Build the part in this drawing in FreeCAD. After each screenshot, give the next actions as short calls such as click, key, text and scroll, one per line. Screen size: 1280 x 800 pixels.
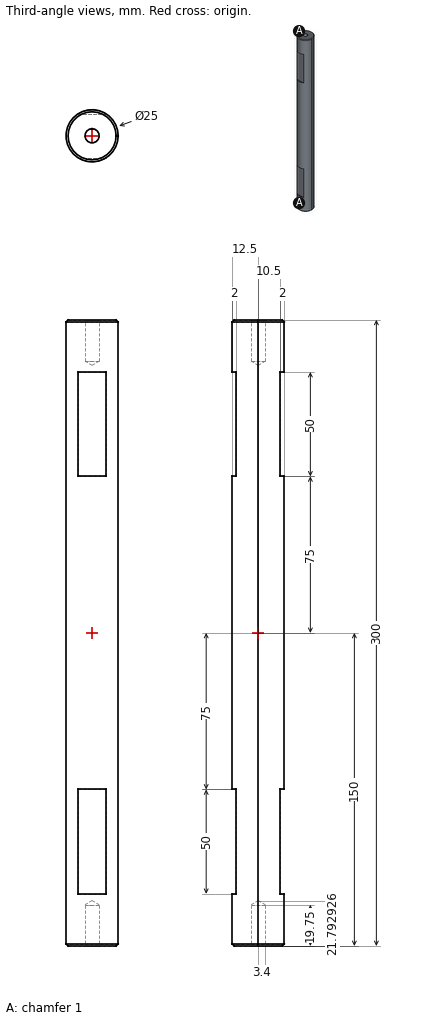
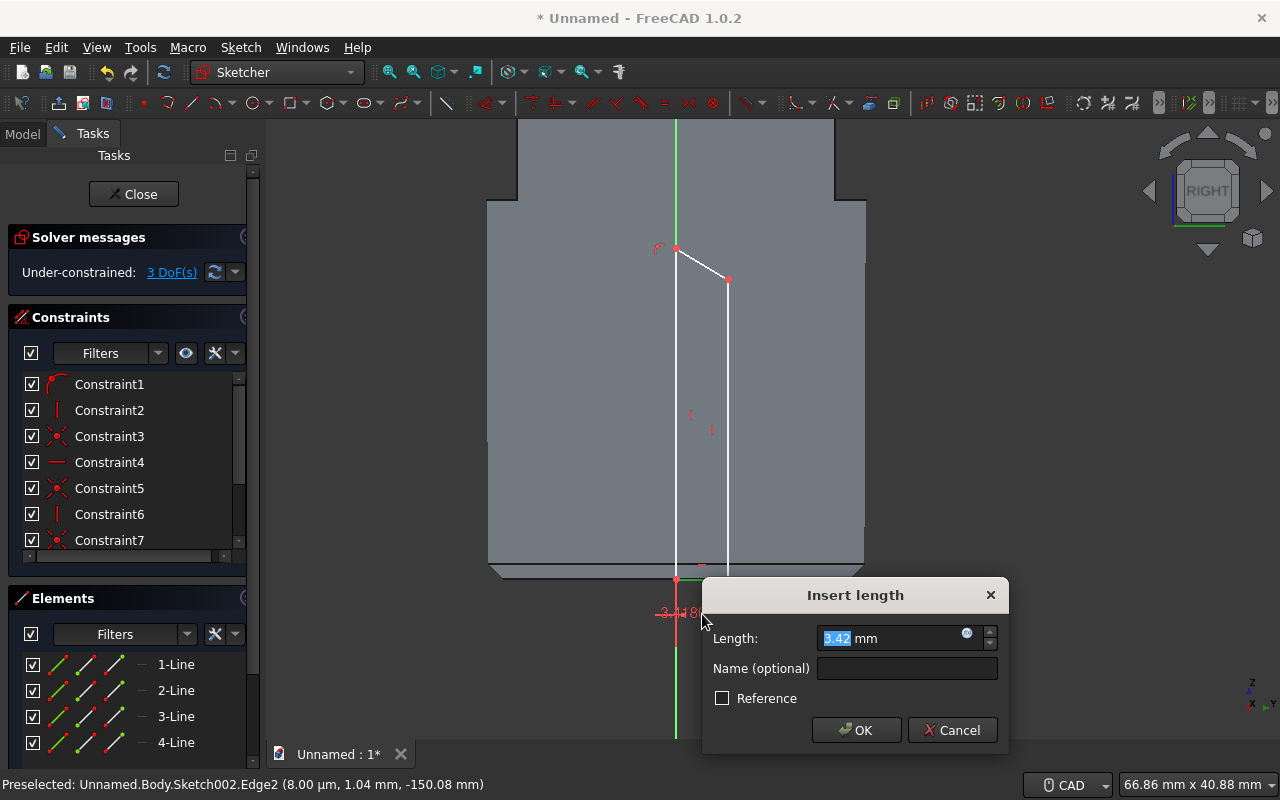
text(3.4)
key(Return)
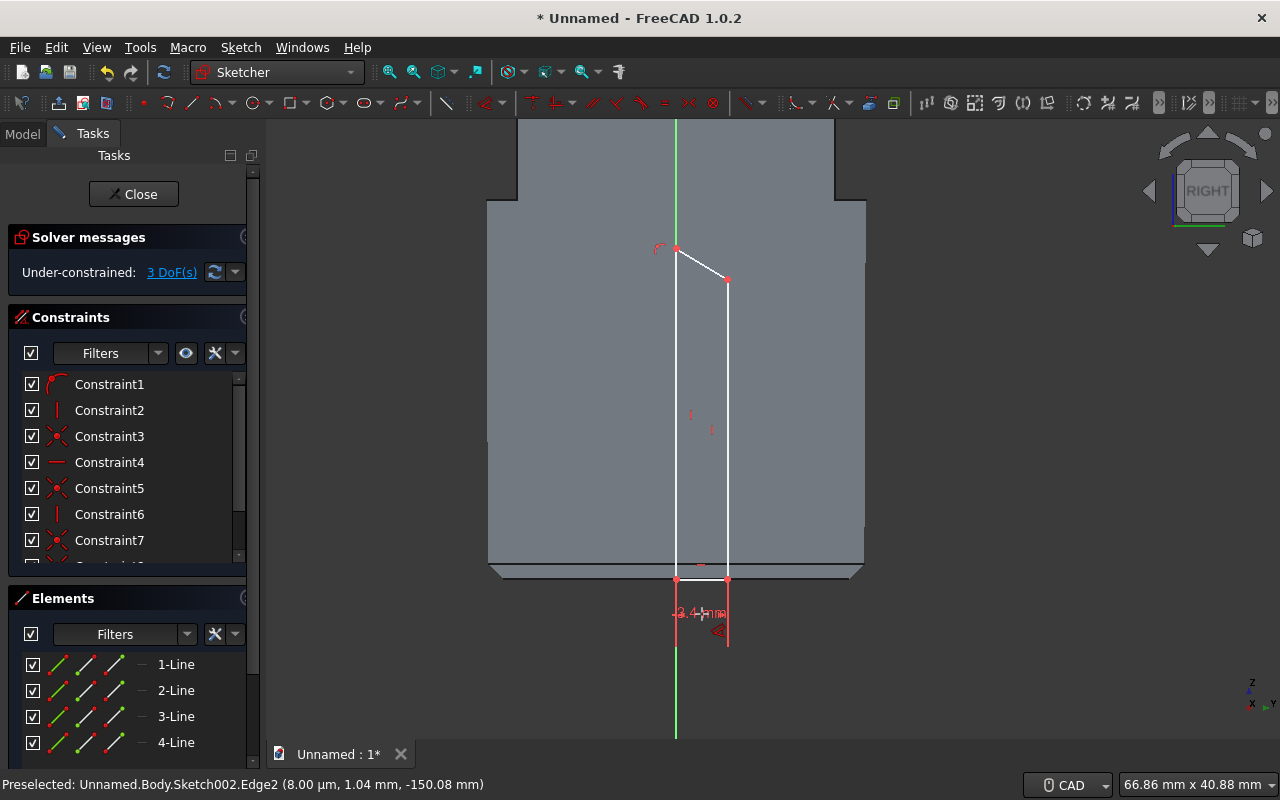
click(676, 580)
click(642, 364)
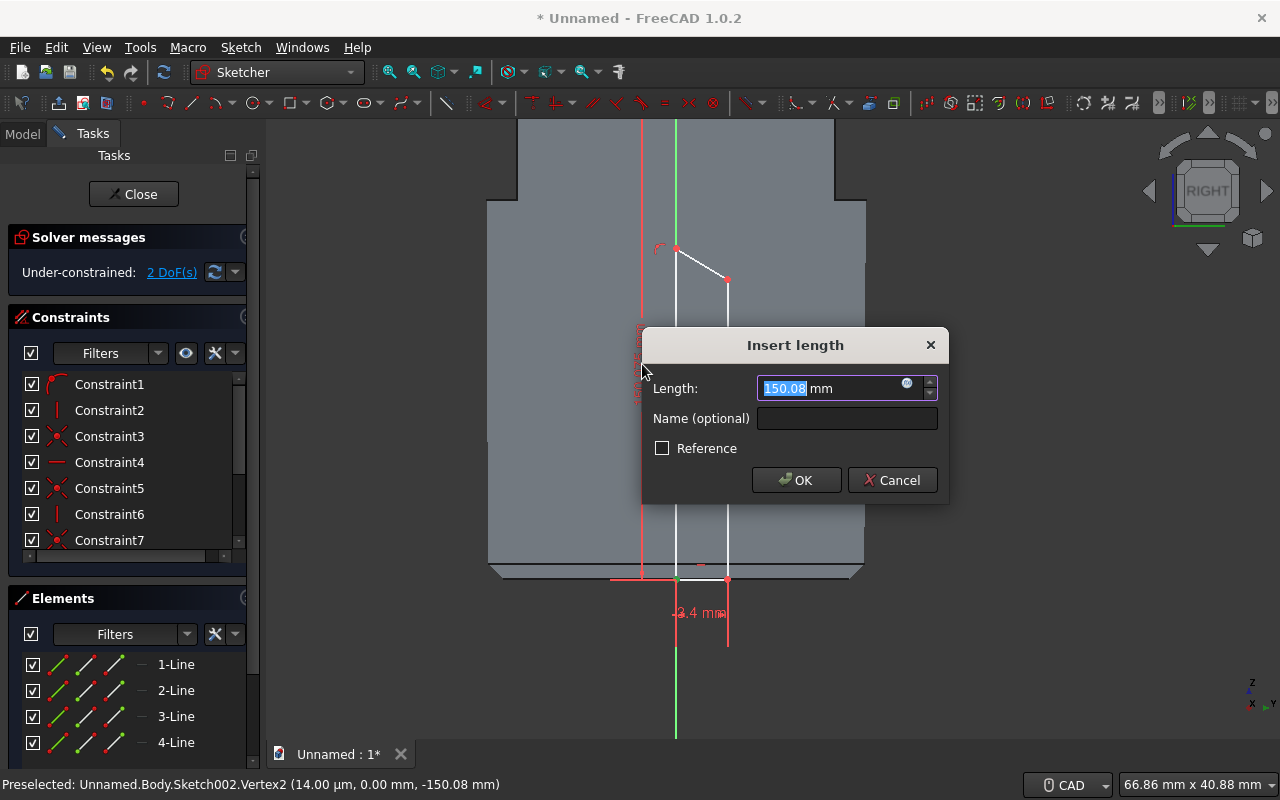
text(150)
key(Return)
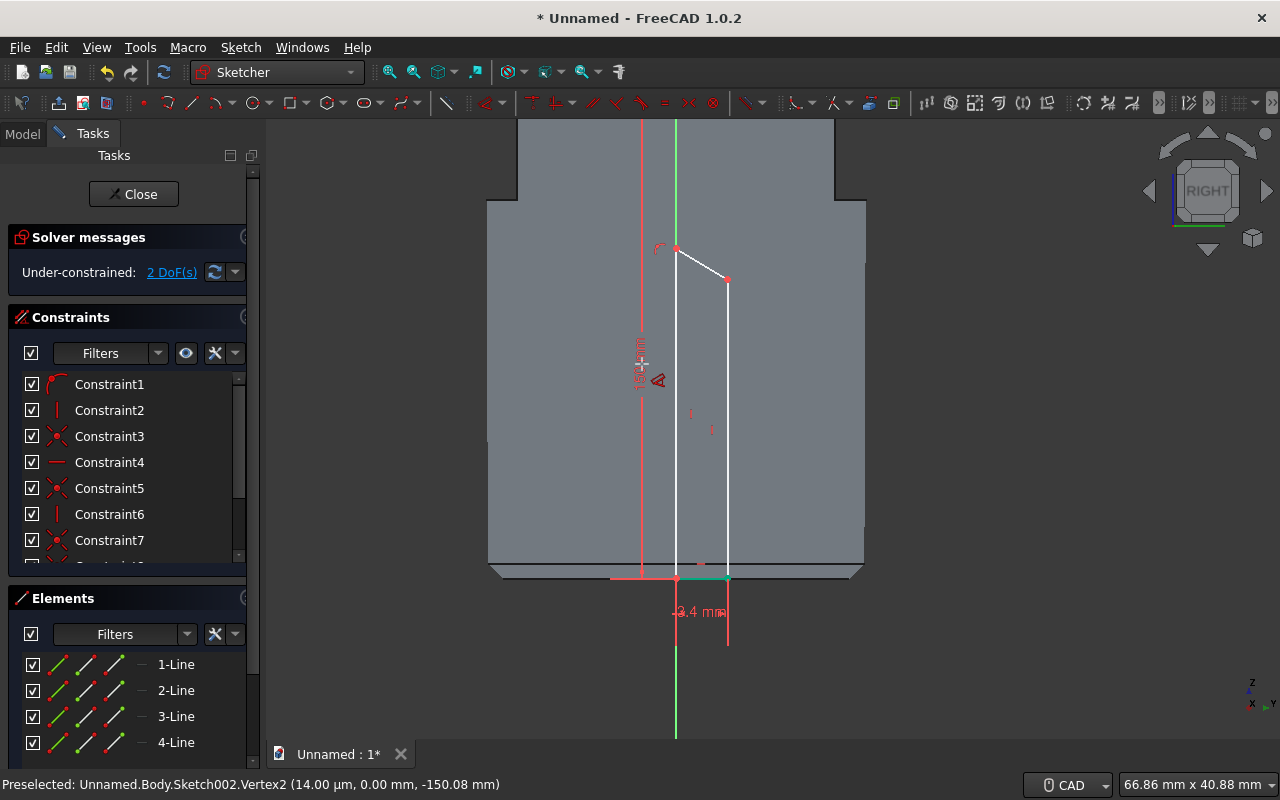
click(728, 489)
click(762, 429)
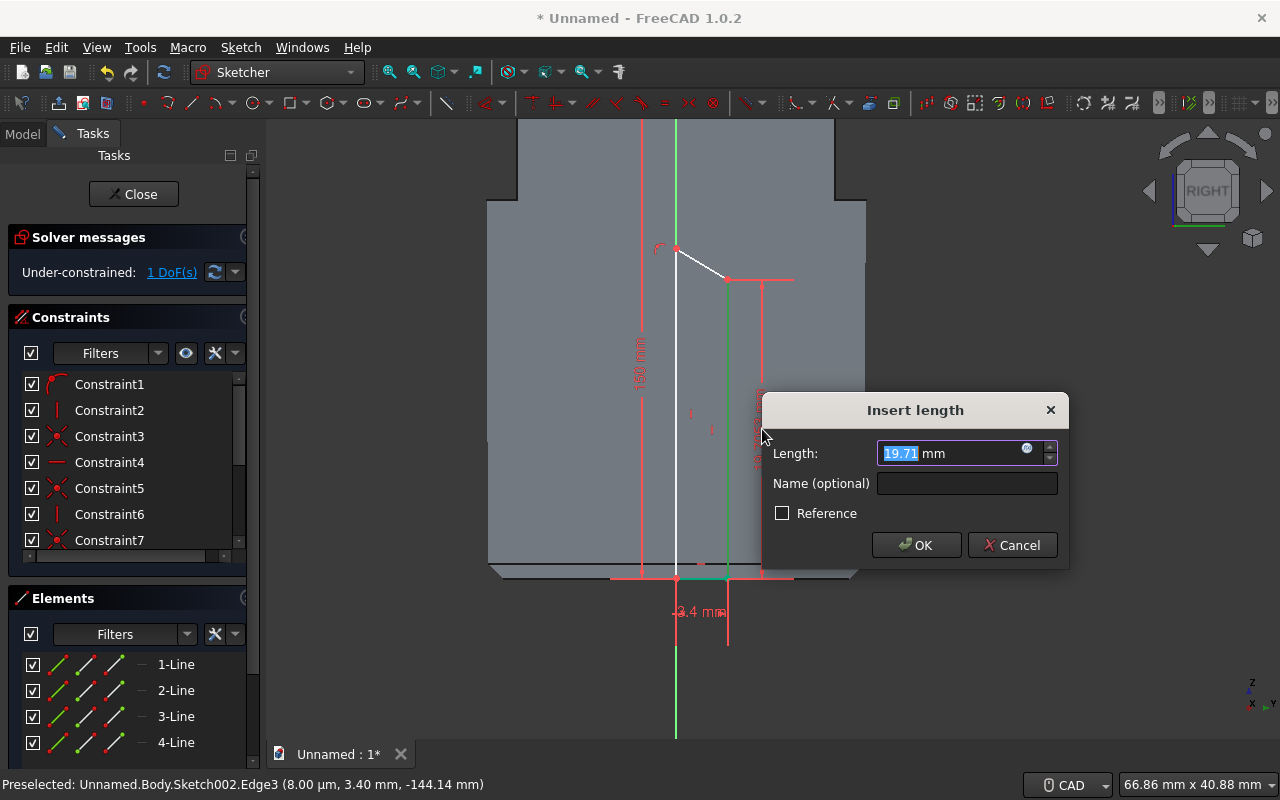
text(19.75)
key(Return)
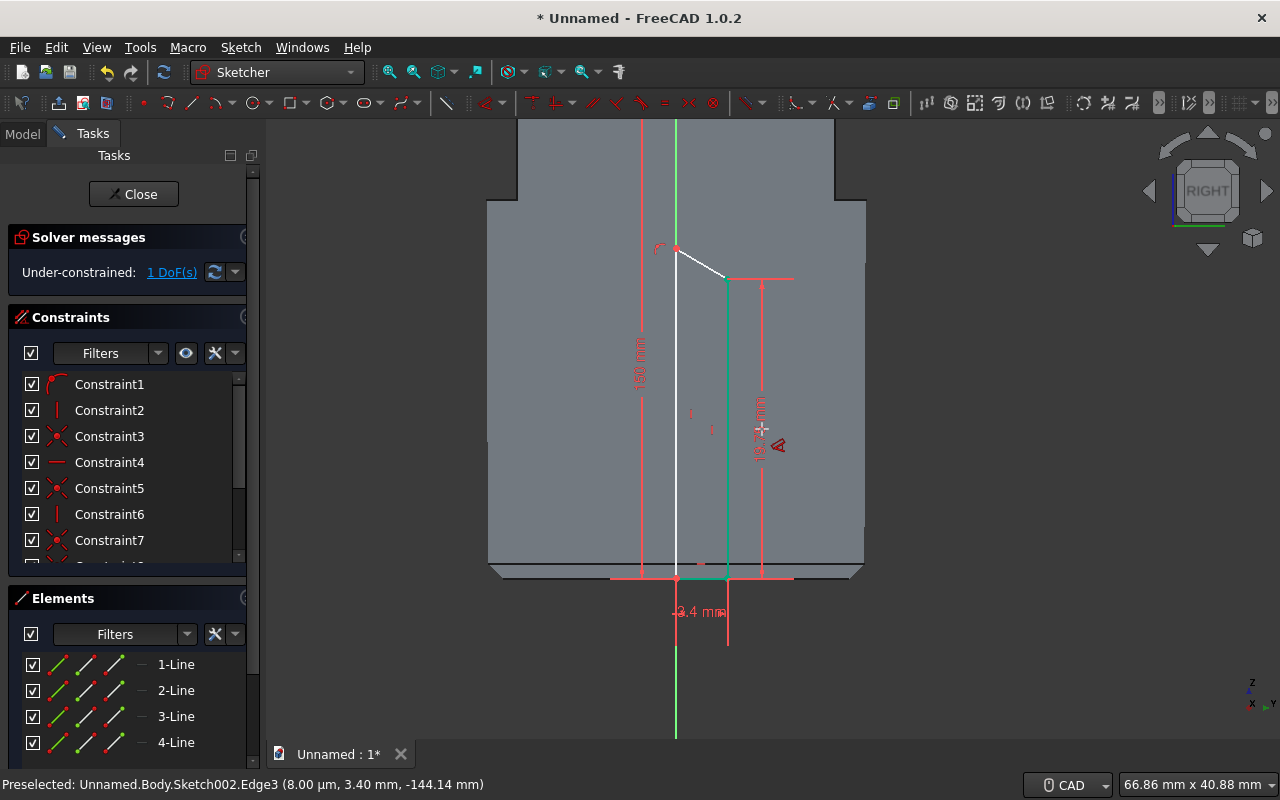
click(676, 348)
click(642, 414)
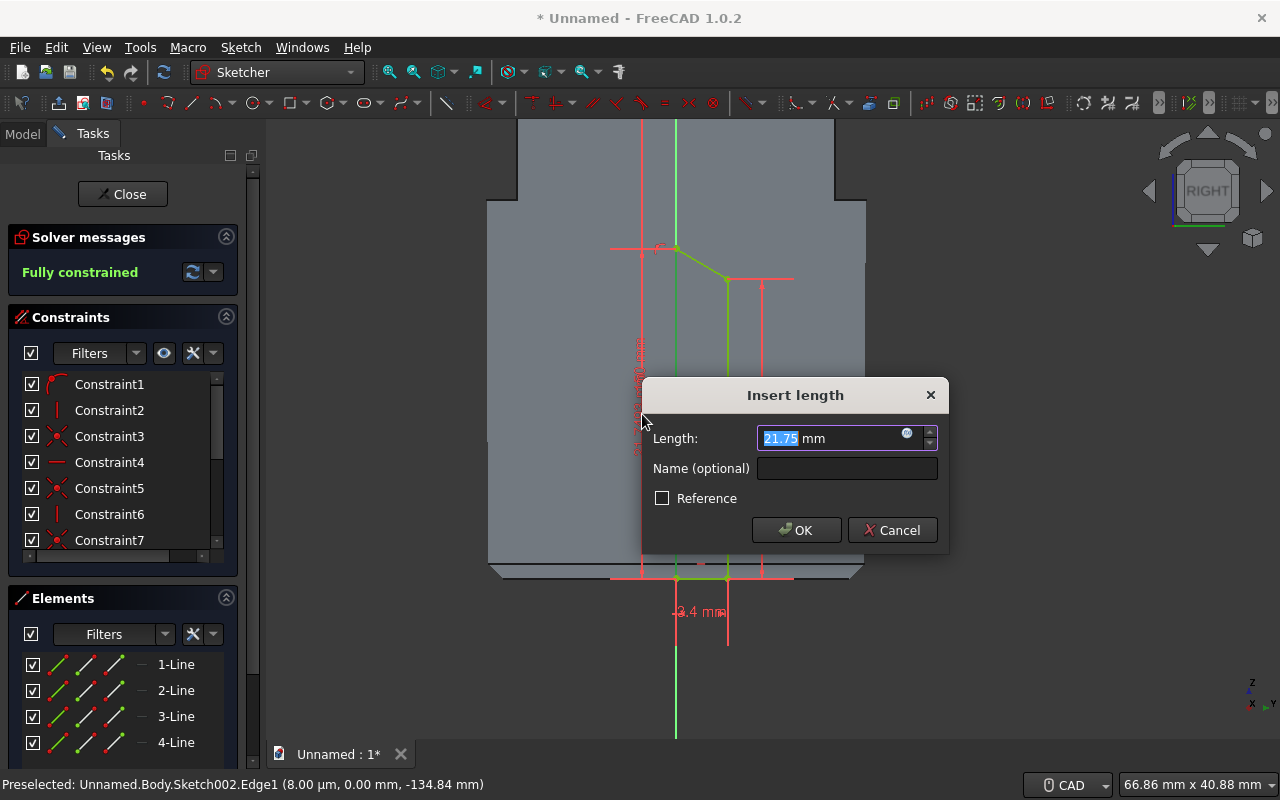
text(21.792926)
key(Return)
key(Escape)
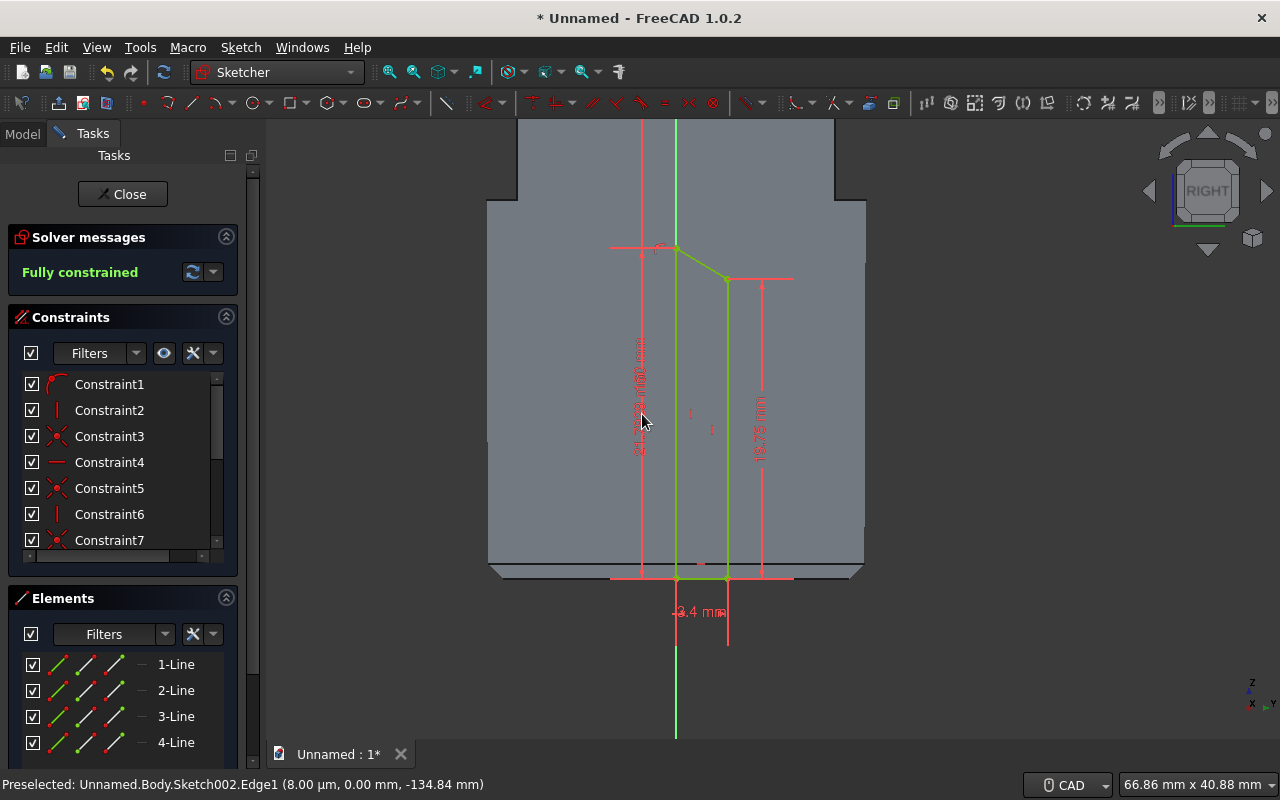
click(123, 194)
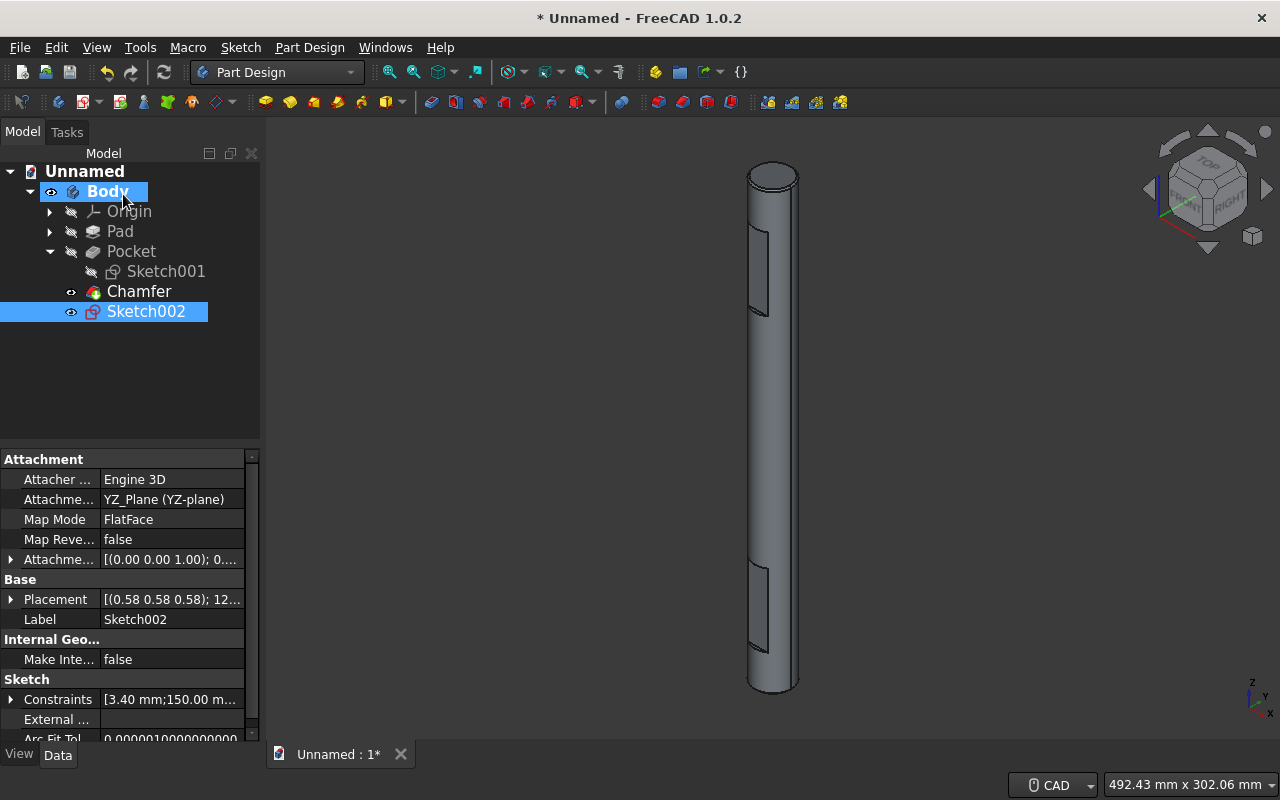
click(480, 102)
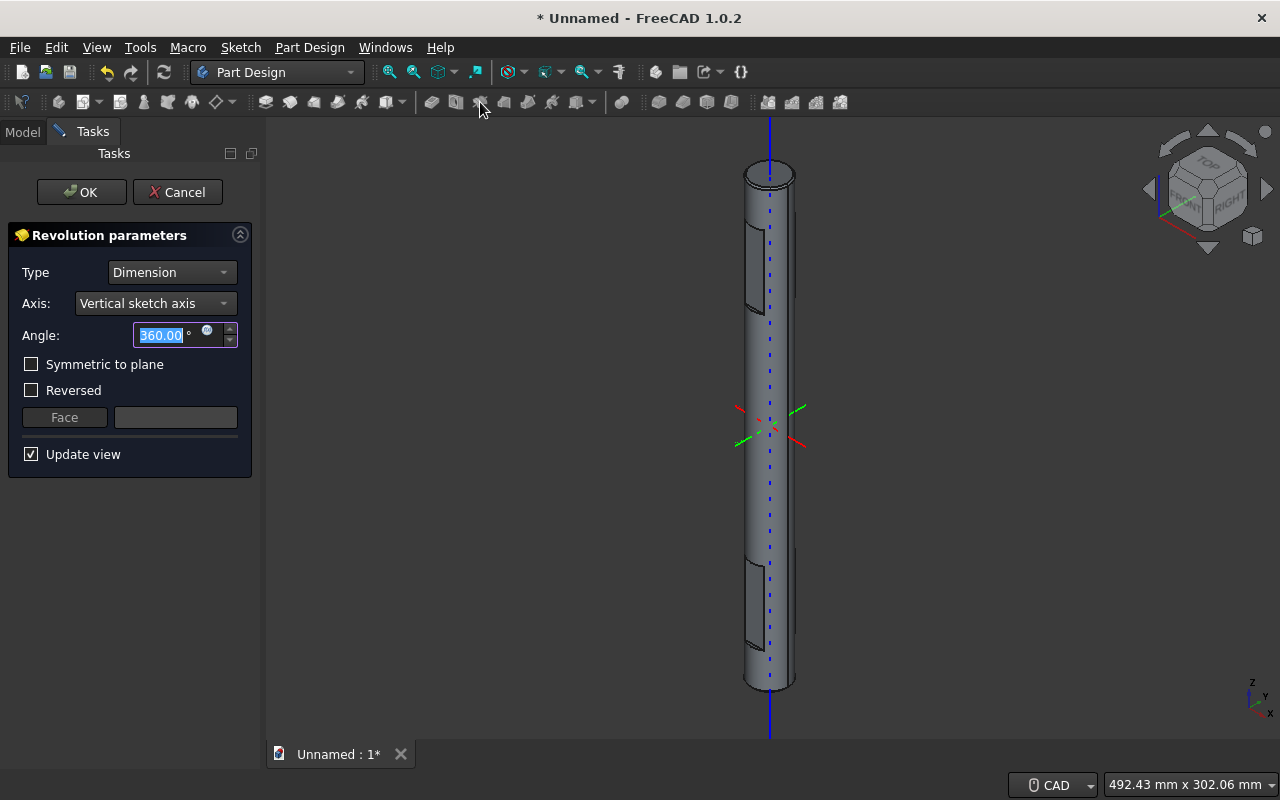
click(82, 192)